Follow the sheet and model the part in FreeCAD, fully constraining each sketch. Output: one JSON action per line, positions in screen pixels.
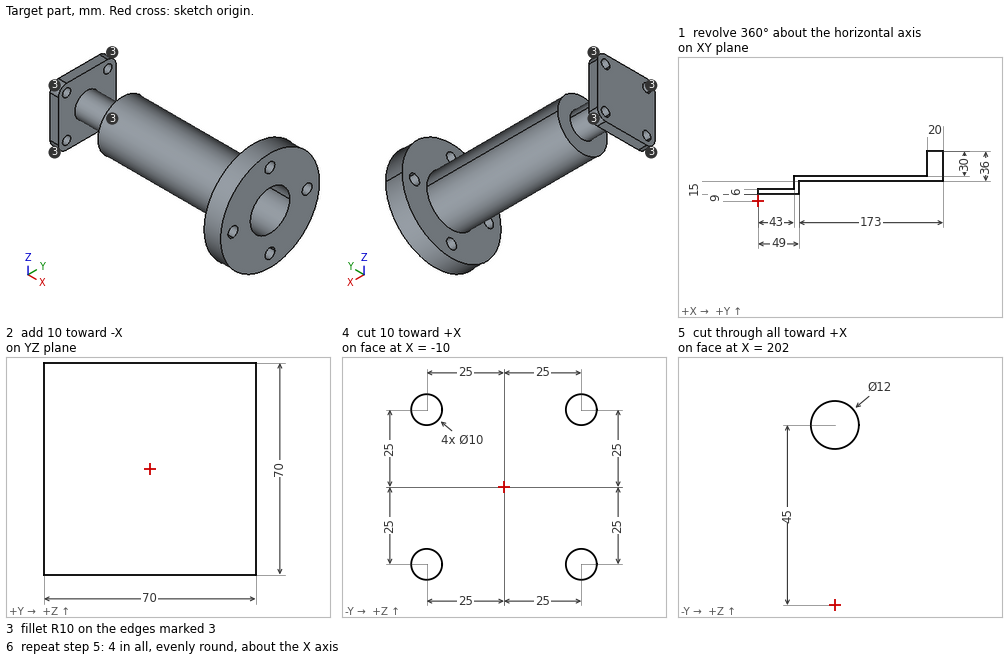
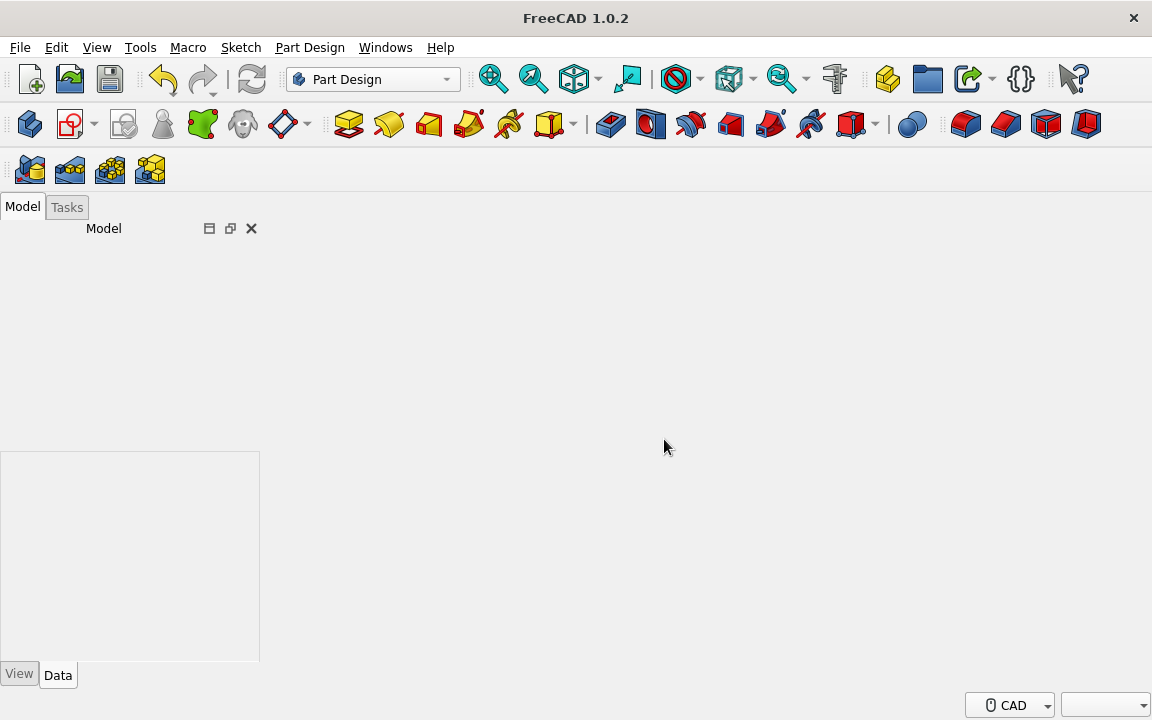
{"action": "left_click", "coordinate": [30, 80]}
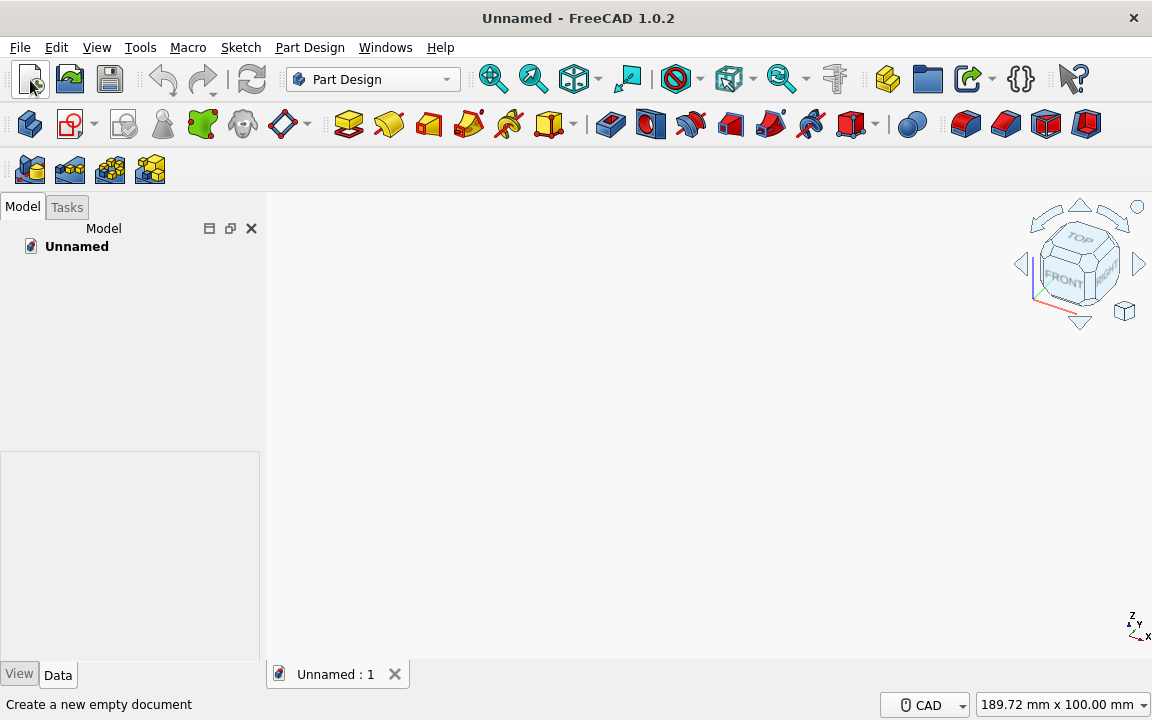
{"action": "left_click", "coordinate": [70, 124]}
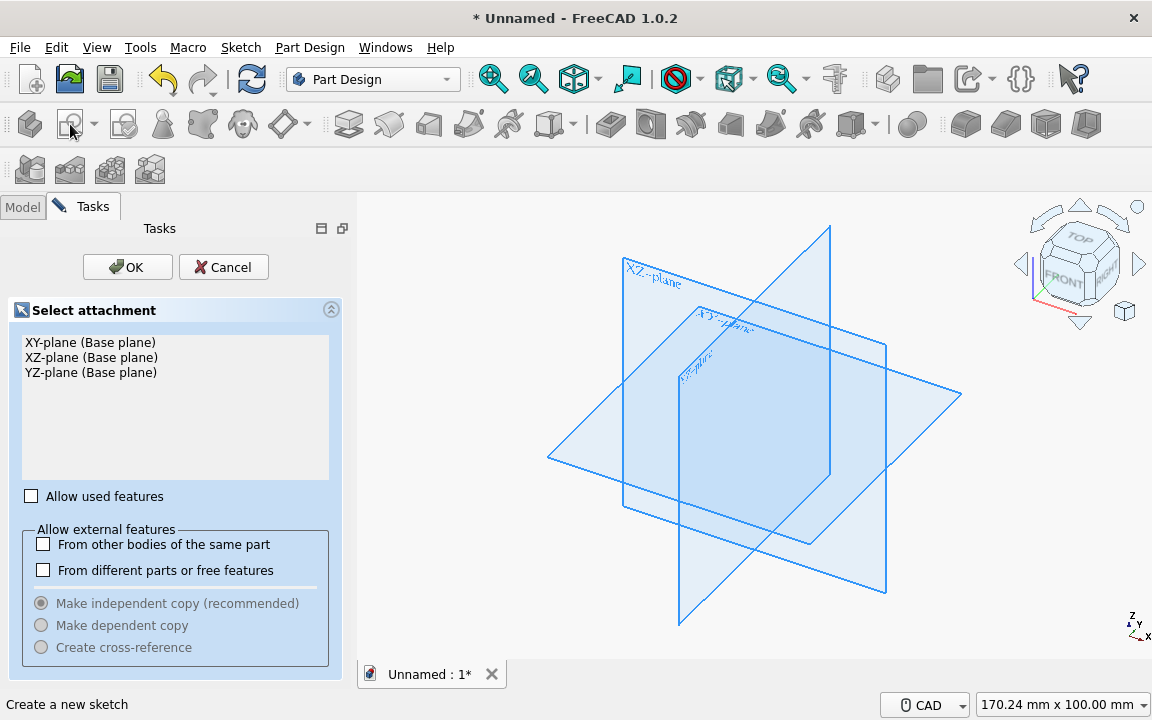
{"action": "left_click", "coordinate": [82, 342]}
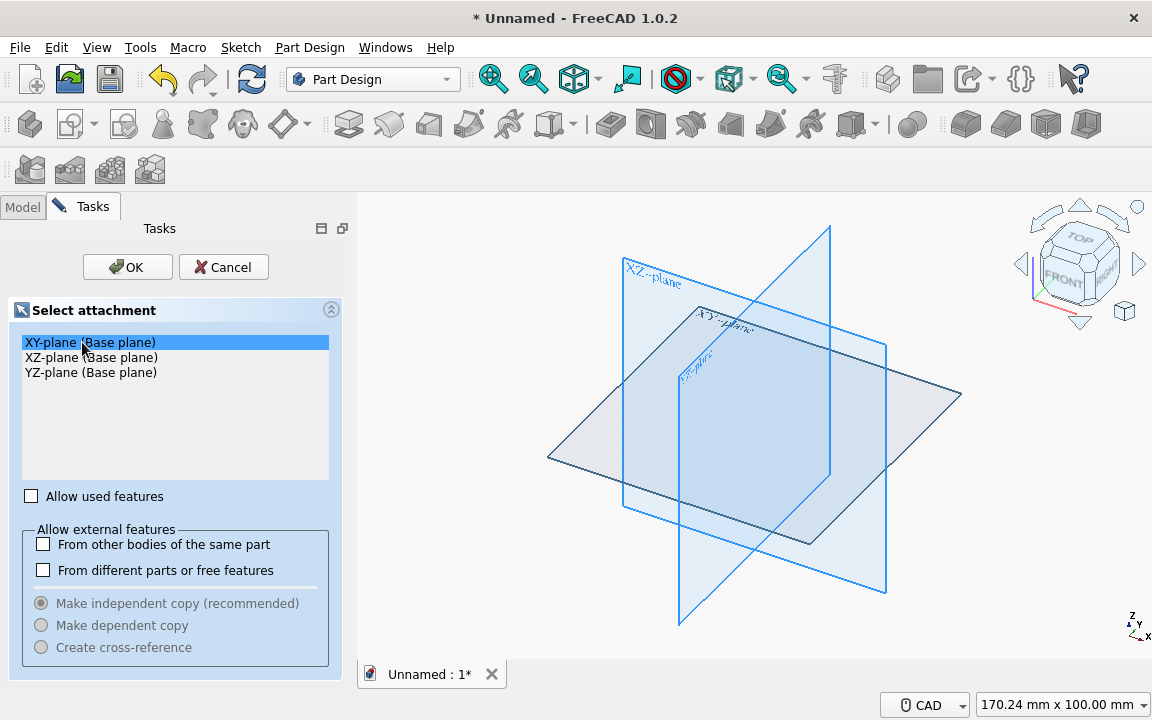
{"action": "left_click", "coordinate": [128, 267]}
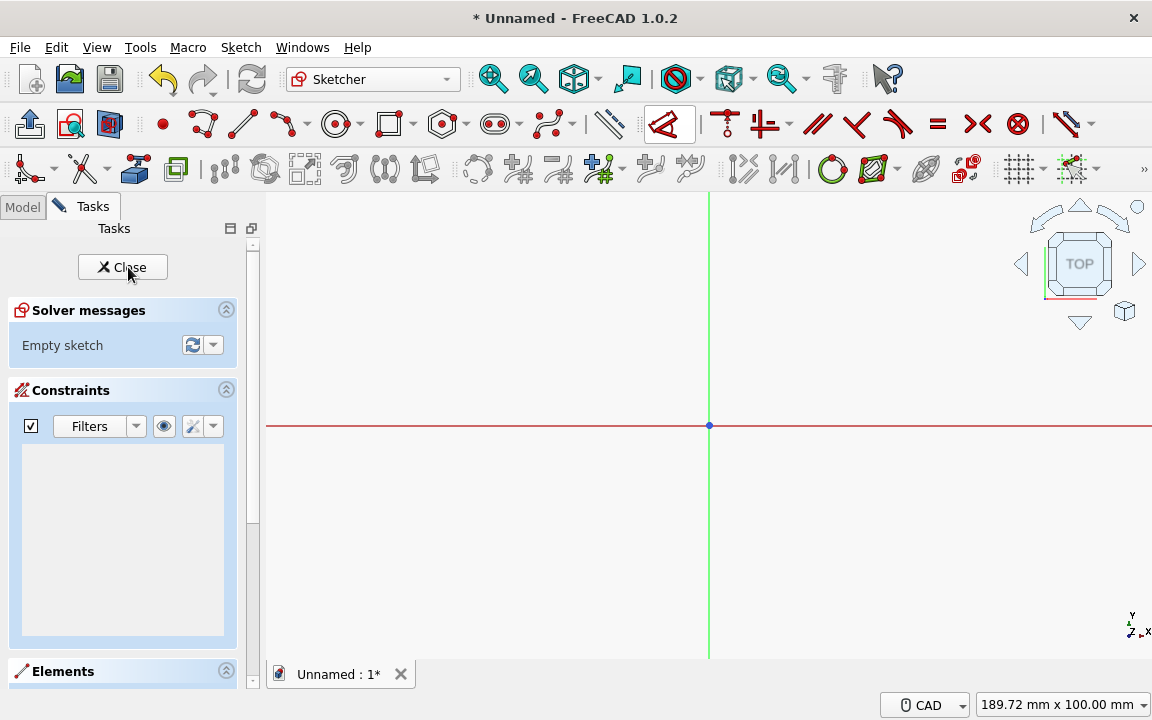
{"action": "scroll", "coordinate": [294, 540], "scroll_direction": "down", "scroll_amount": 4}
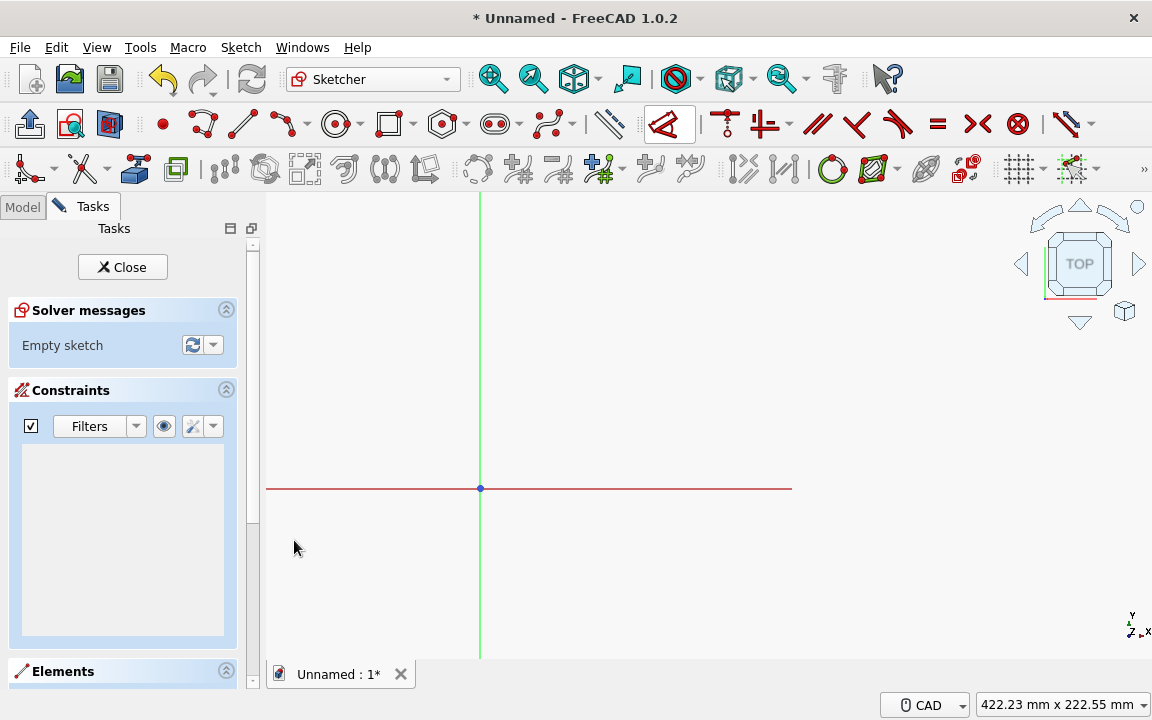
{"action": "left_click", "coordinate": [204, 124]}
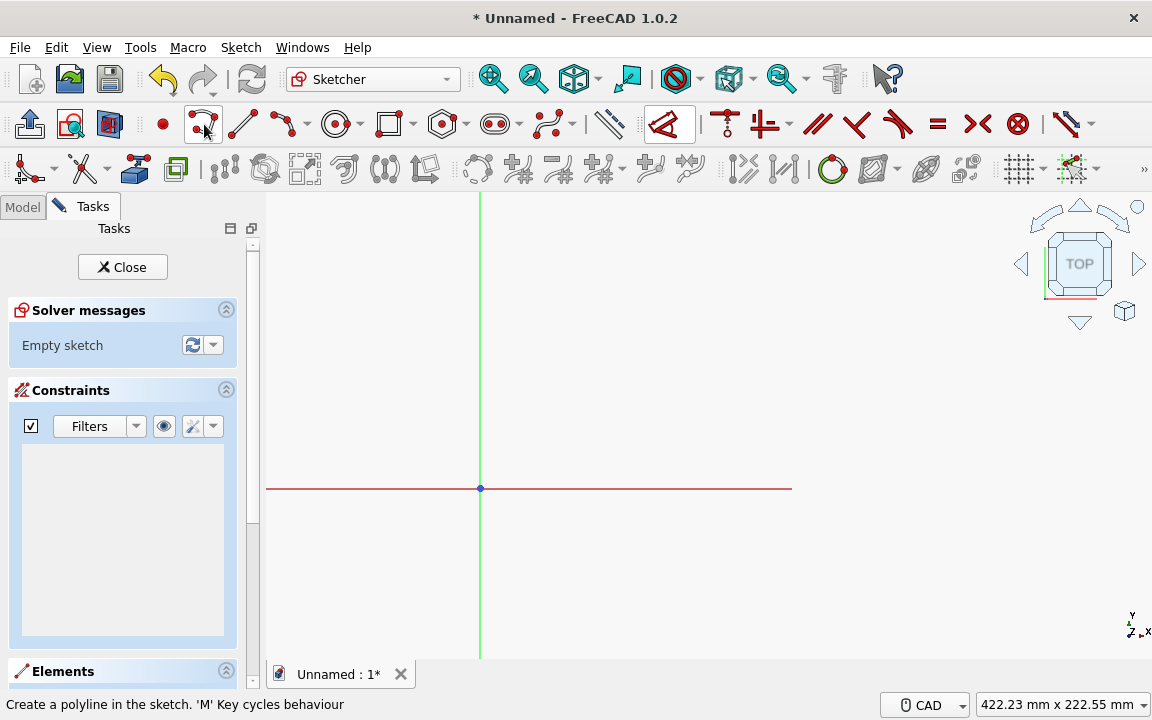
{"action": "left_click", "coordinate": [480, 470]}
{"action": "left_click", "coordinate": [583, 470]}
{"action": "left_click", "coordinate": [583, 439]}
{"action": "left_click", "coordinate": [946, 439]}
{"action": "left_click", "coordinate": [946, 363]}
{"action": "left_click", "coordinate": [904, 363]}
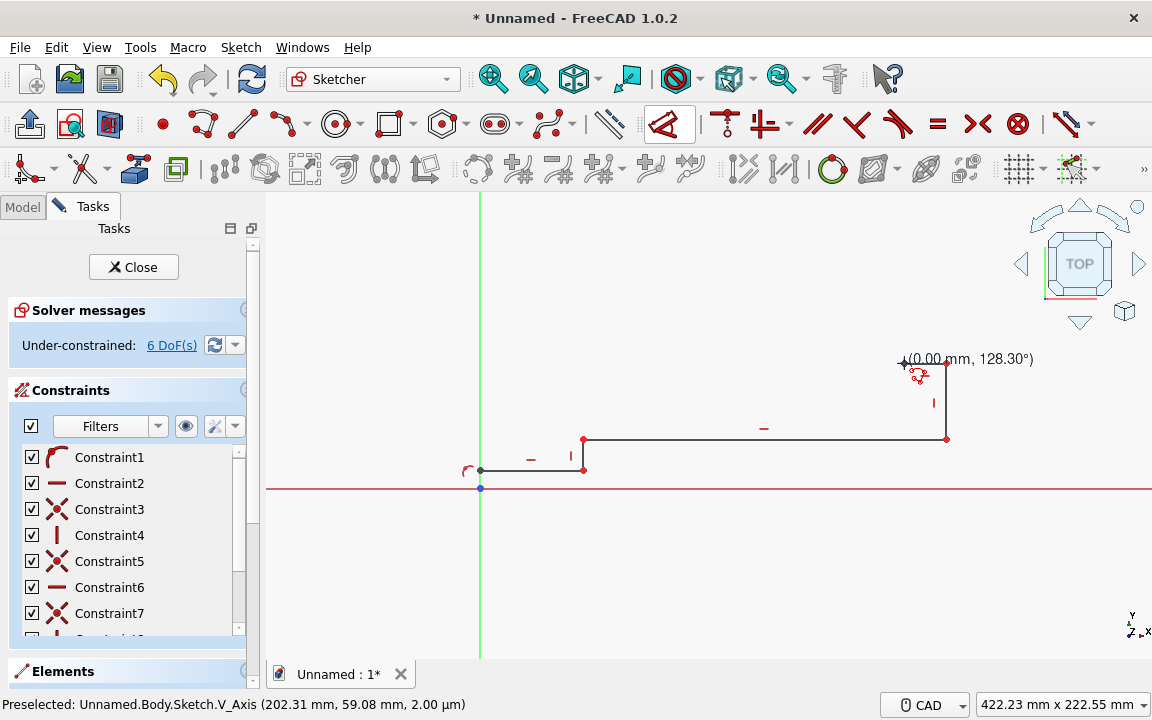
{"action": "scroll", "coordinate": [904, 426], "scroll_direction": "up", "scroll_amount": 2}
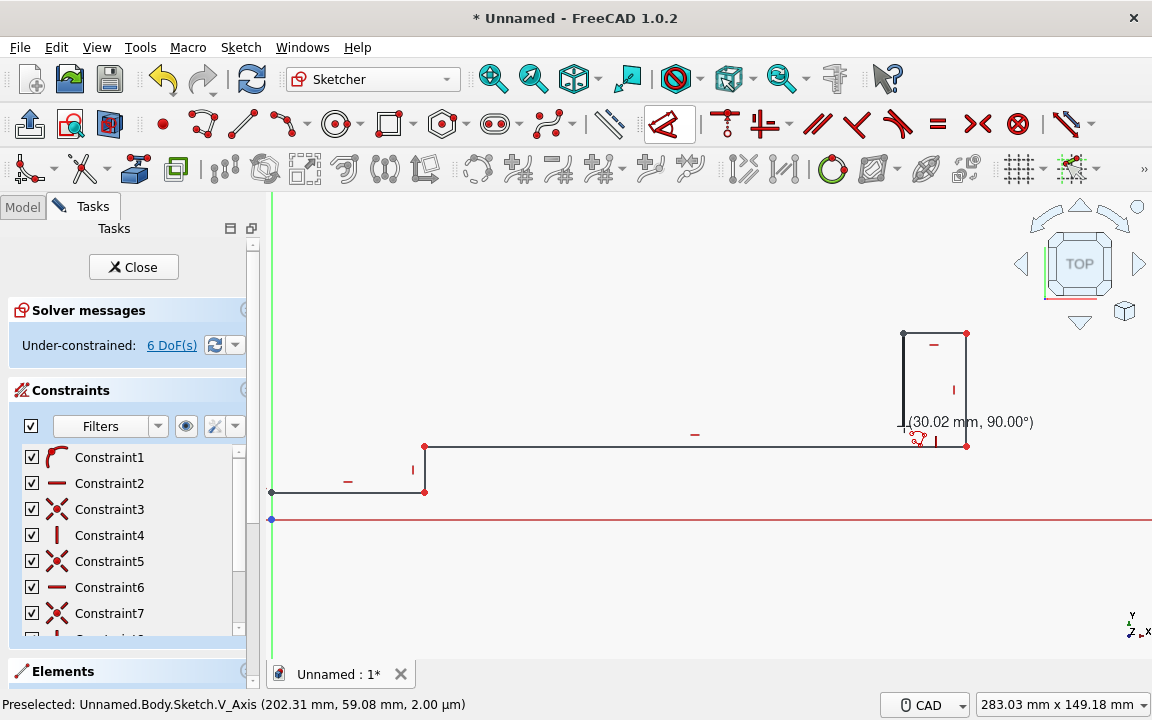
{"action": "left_click", "coordinate": [904, 426]}
{"action": "left_click", "coordinate": [406, 426]}
{"action": "left_click", "coordinate": [406, 473]}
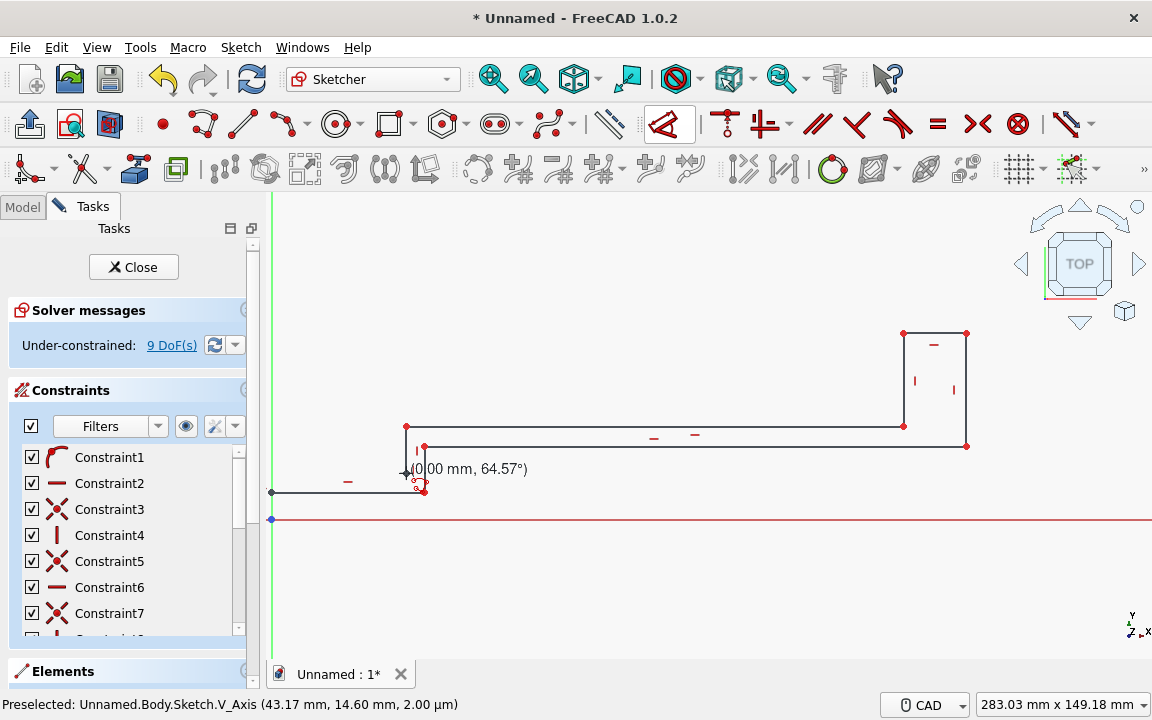
{"action": "scroll", "coordinate": [684, 425], "scroll_direction": "down", "scroll_amount": 2}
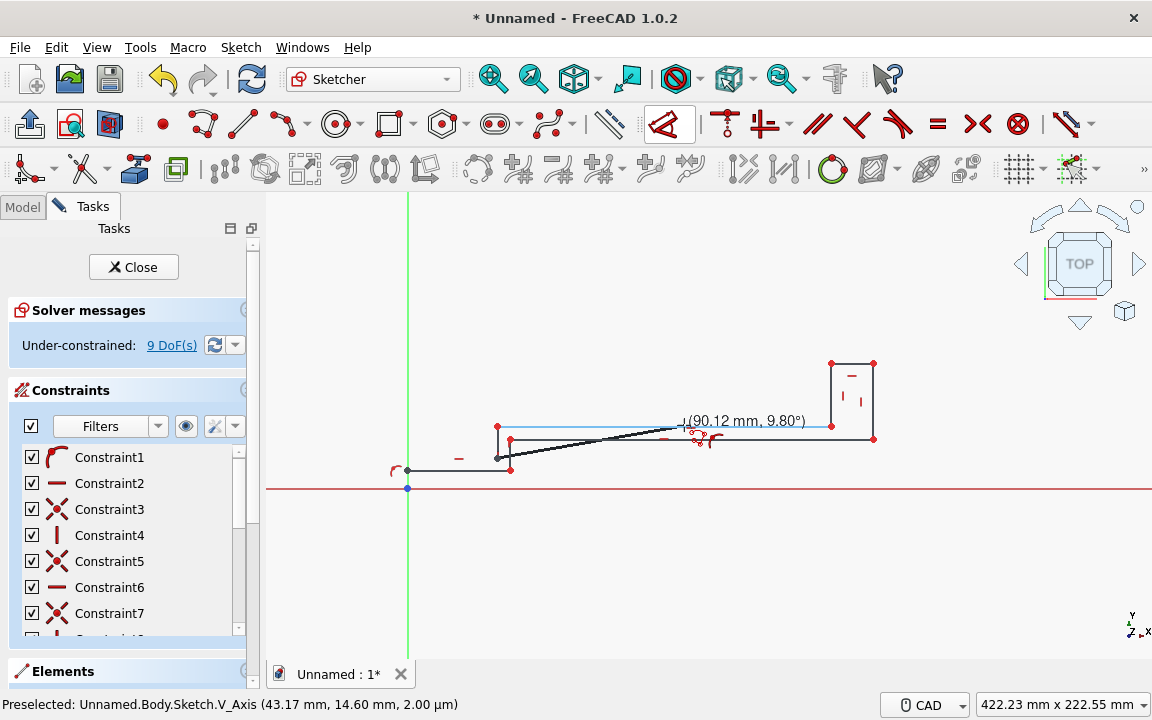
{"action": "scroll", "coordinate": [408, 457], "scroll_direction": "up", "scroll_amount": 2}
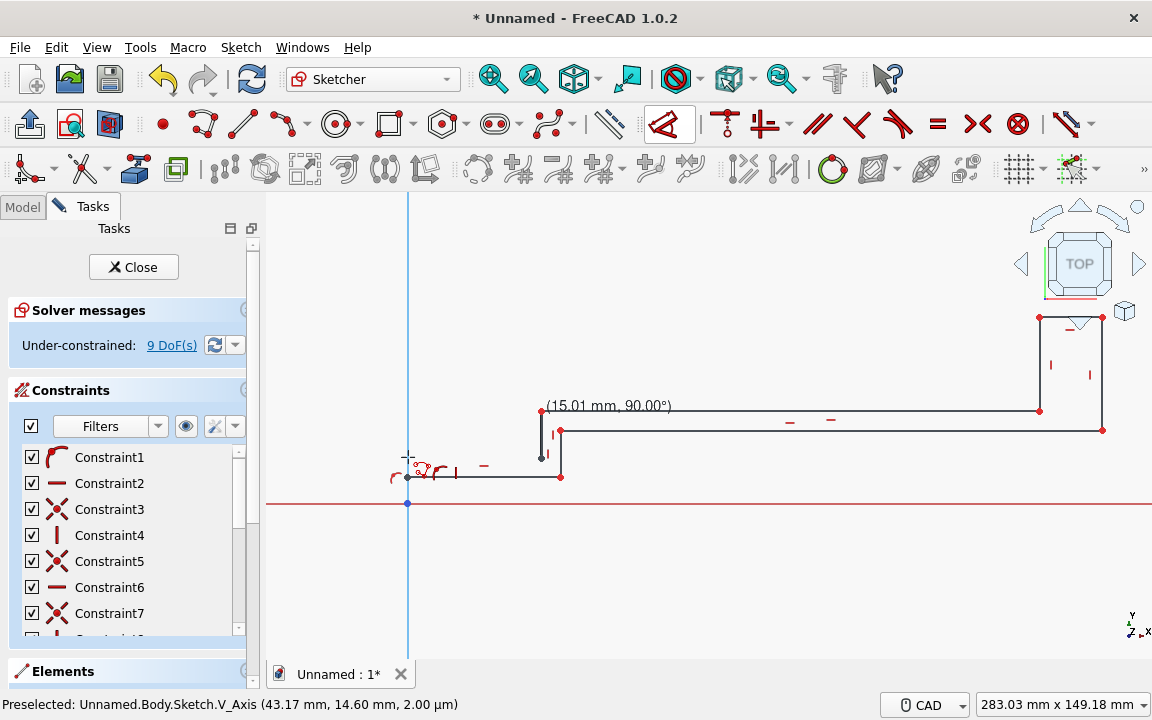
{"action": "left_click", "coordinate": [417, 457]}
{"action": "left_click", "coordinate": [408, 477]}
{"action": "key", "text": "Escape"}
{"action": "key", "text": "Escape"}